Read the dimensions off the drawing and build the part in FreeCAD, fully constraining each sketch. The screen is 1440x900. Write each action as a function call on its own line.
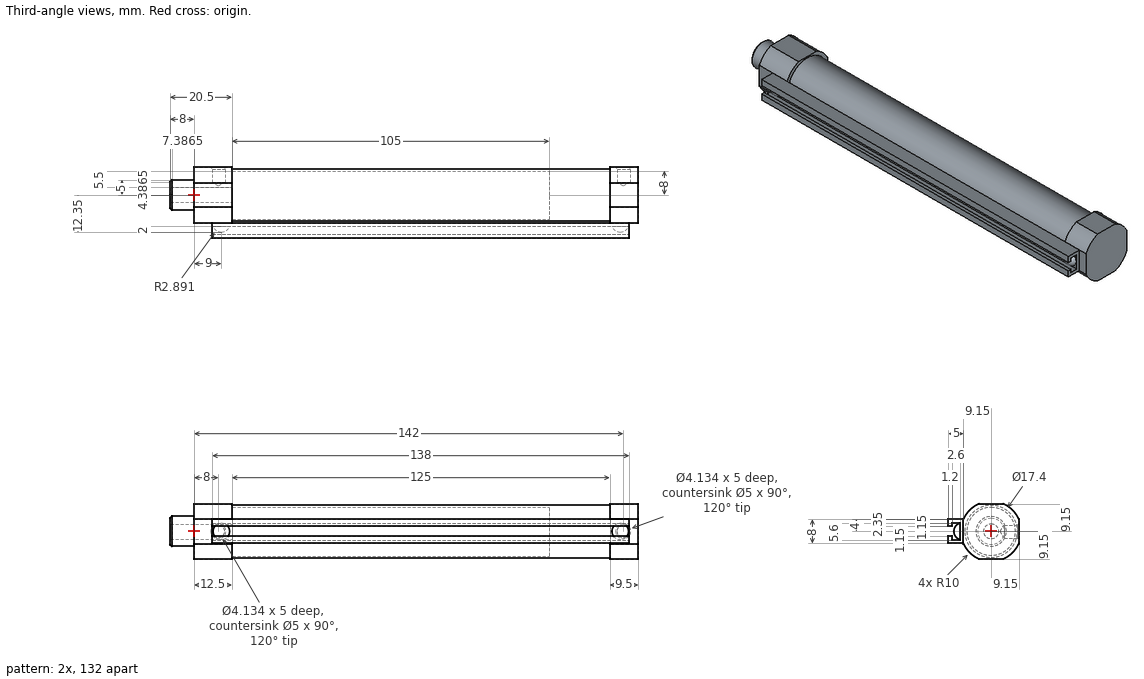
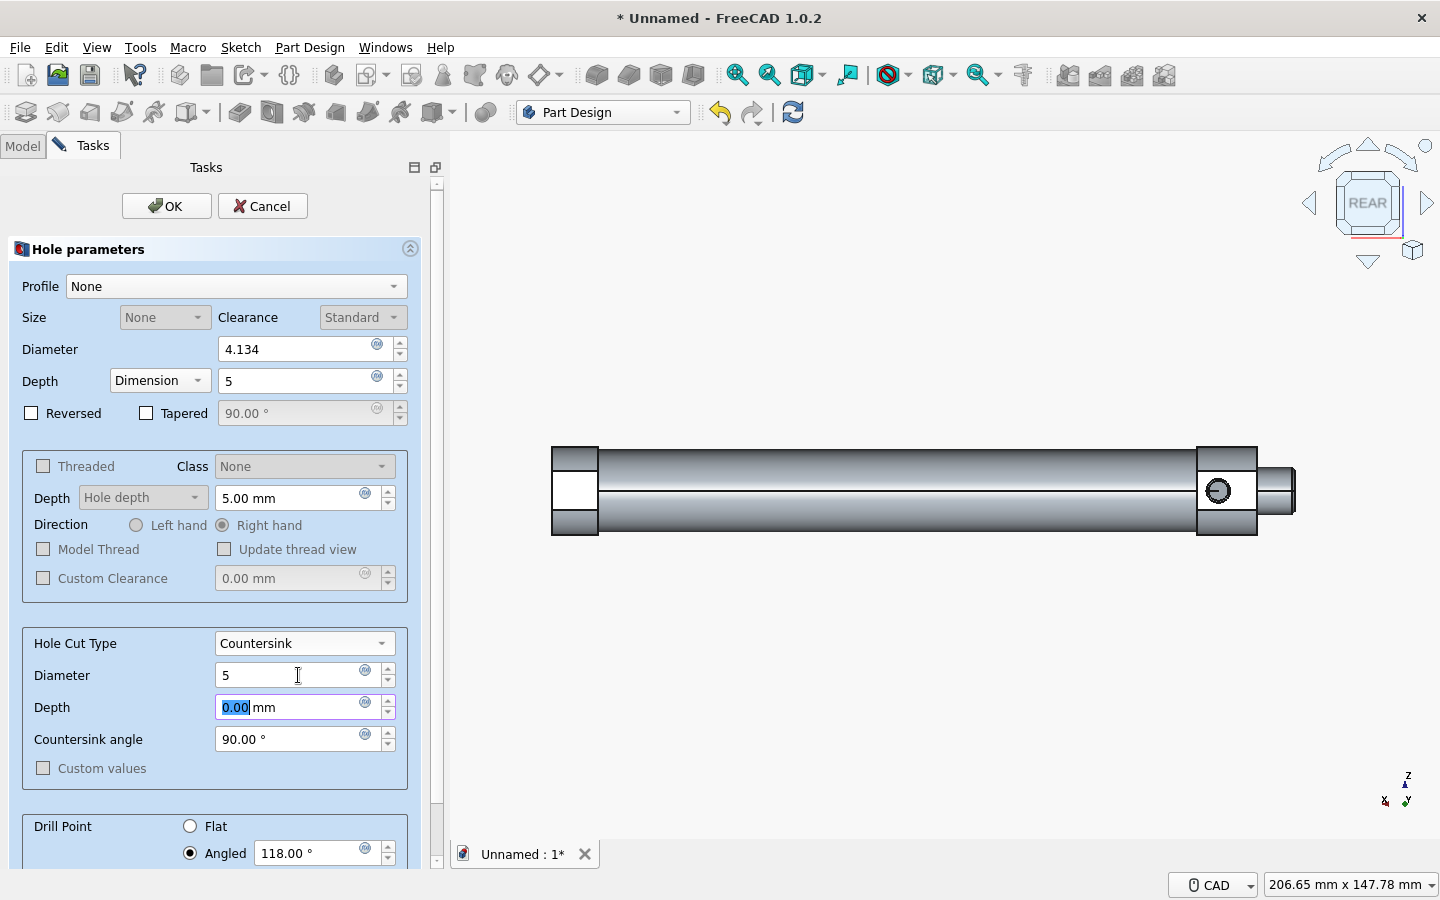
triple_click(317, 853)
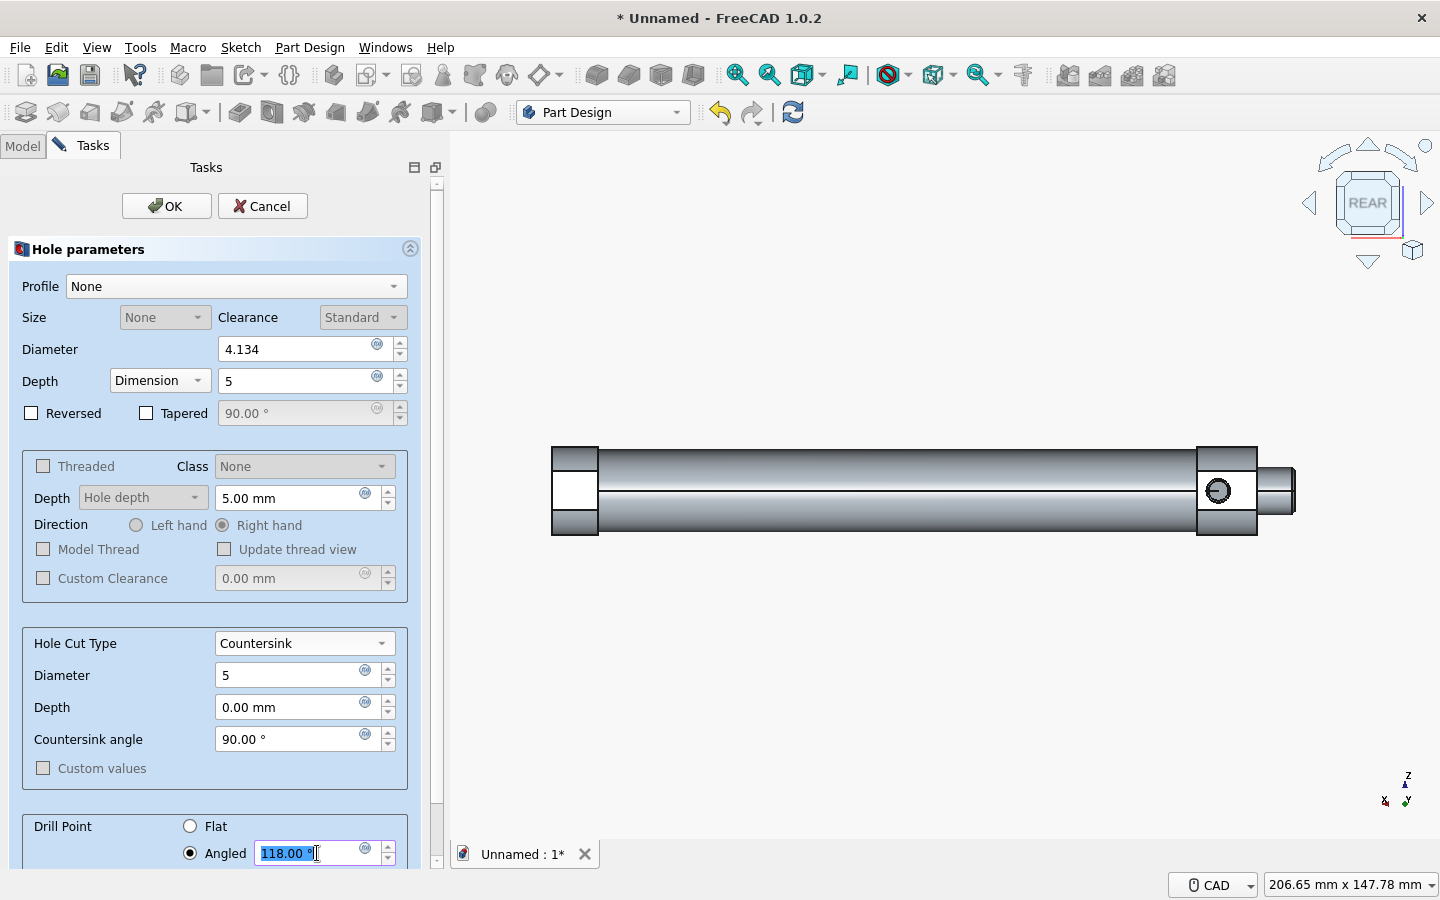
text(120)
key(Tab)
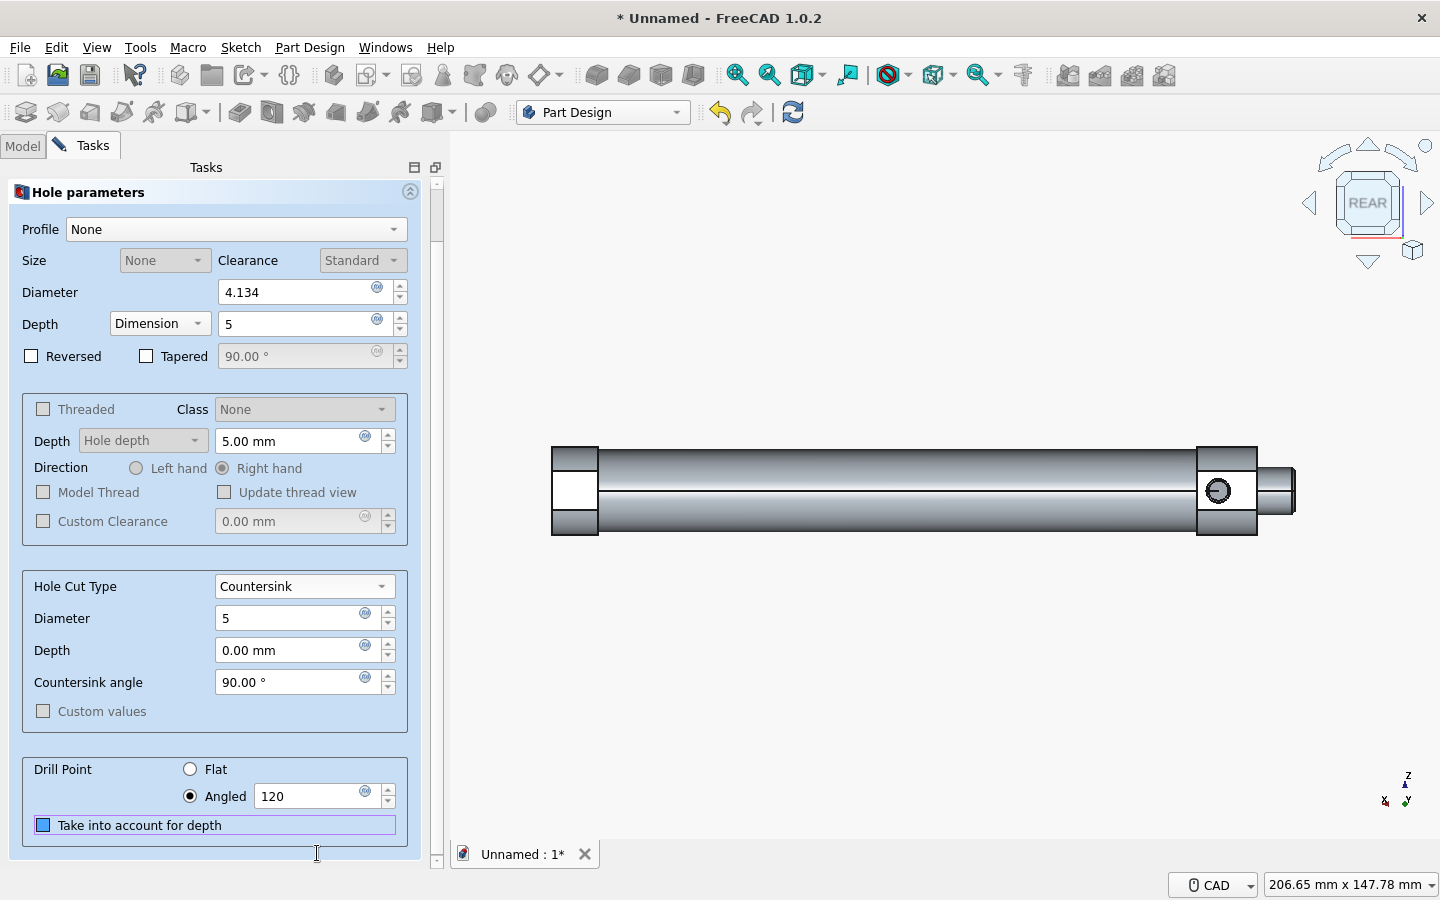
scroll(437, 522, up, 2)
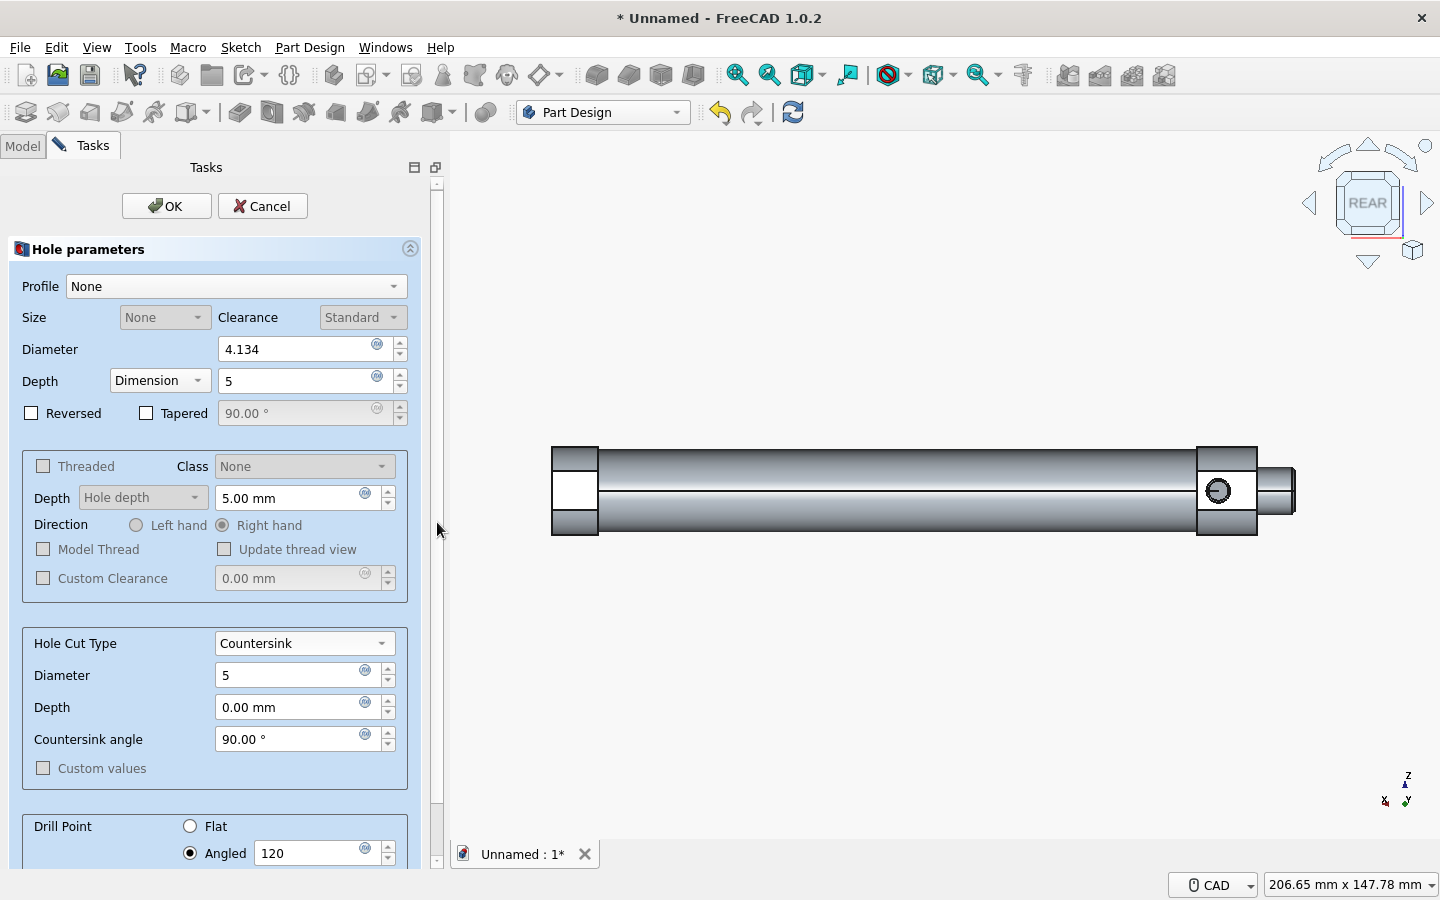
click(167, 206)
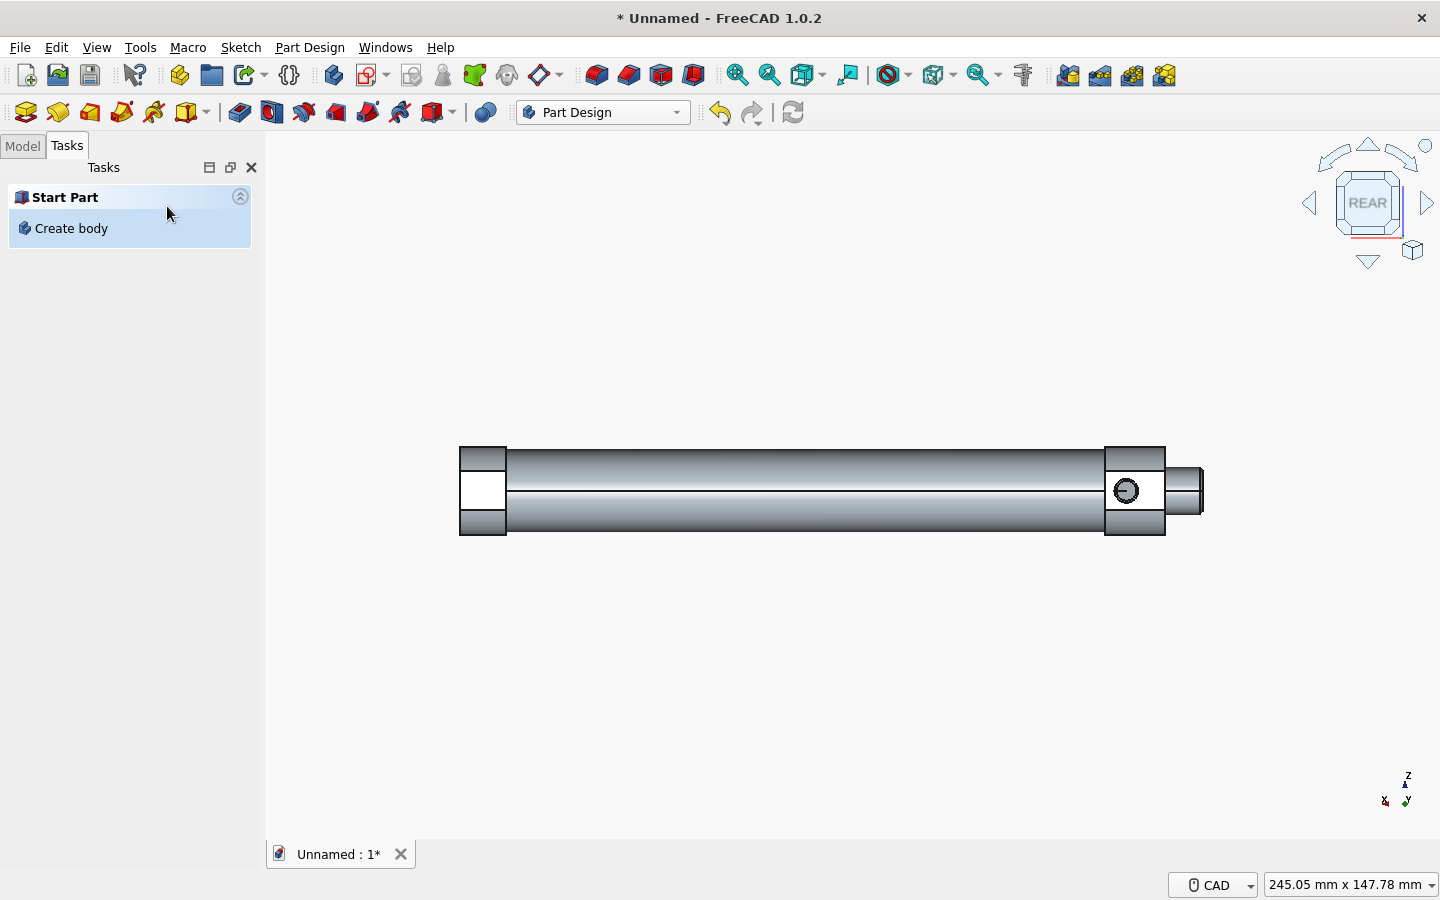
click(1152, 484)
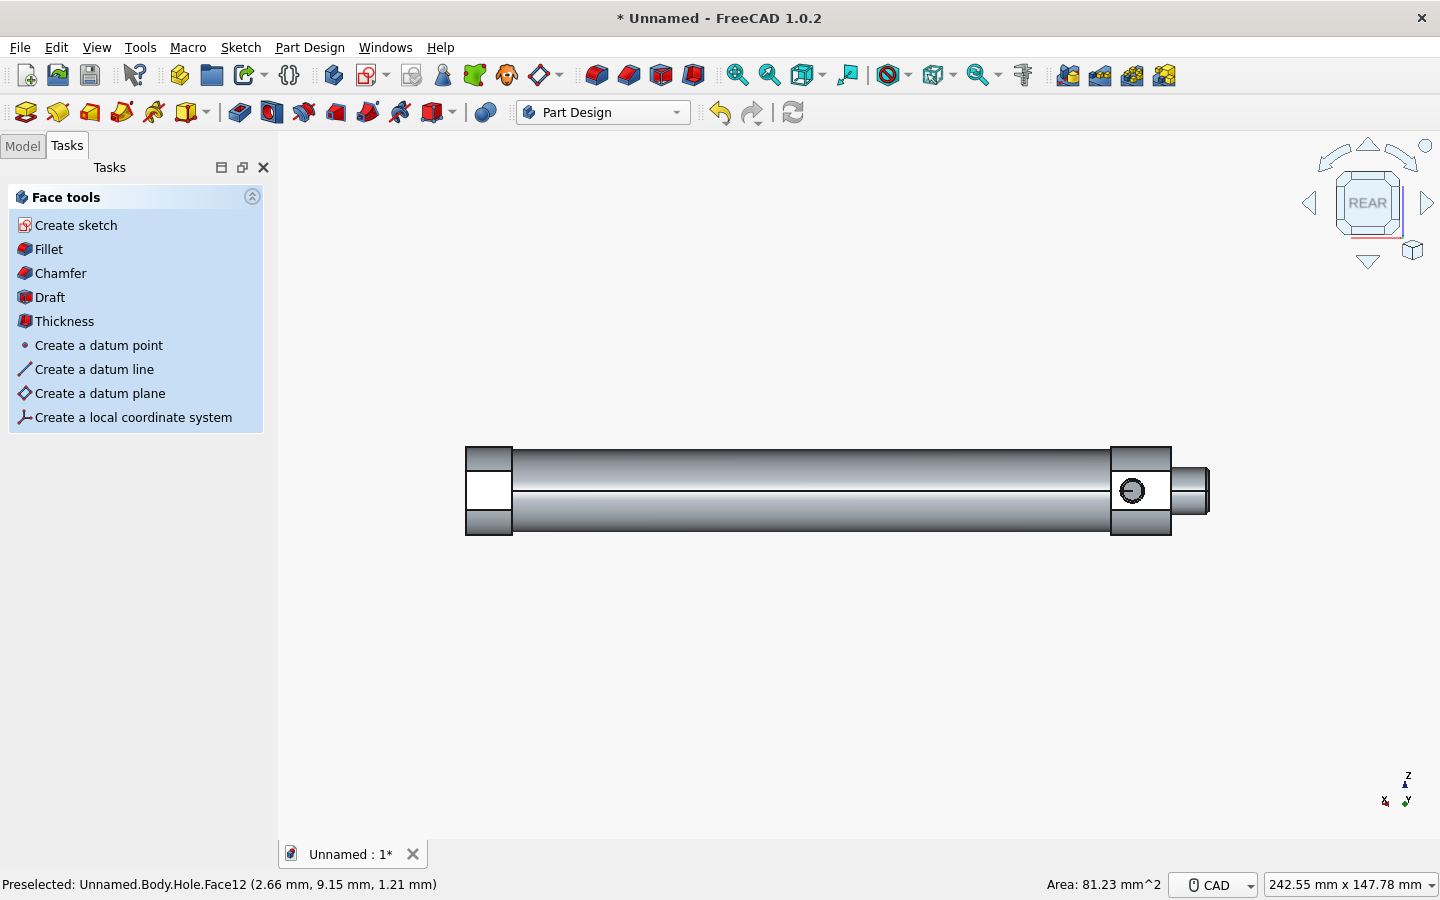
click(366, 76)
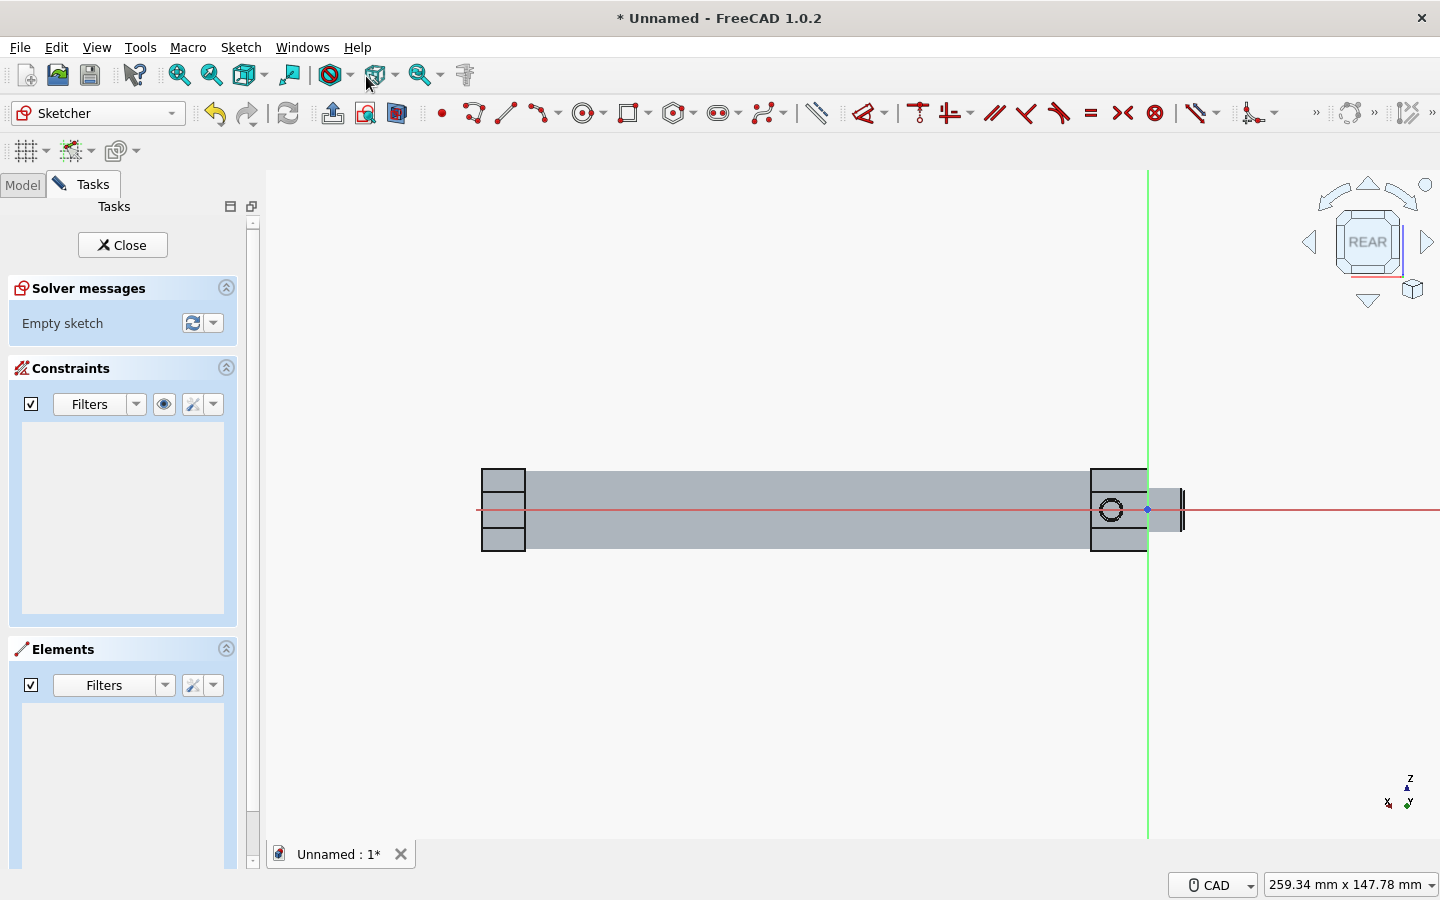
scroll(490, 510, up, 15)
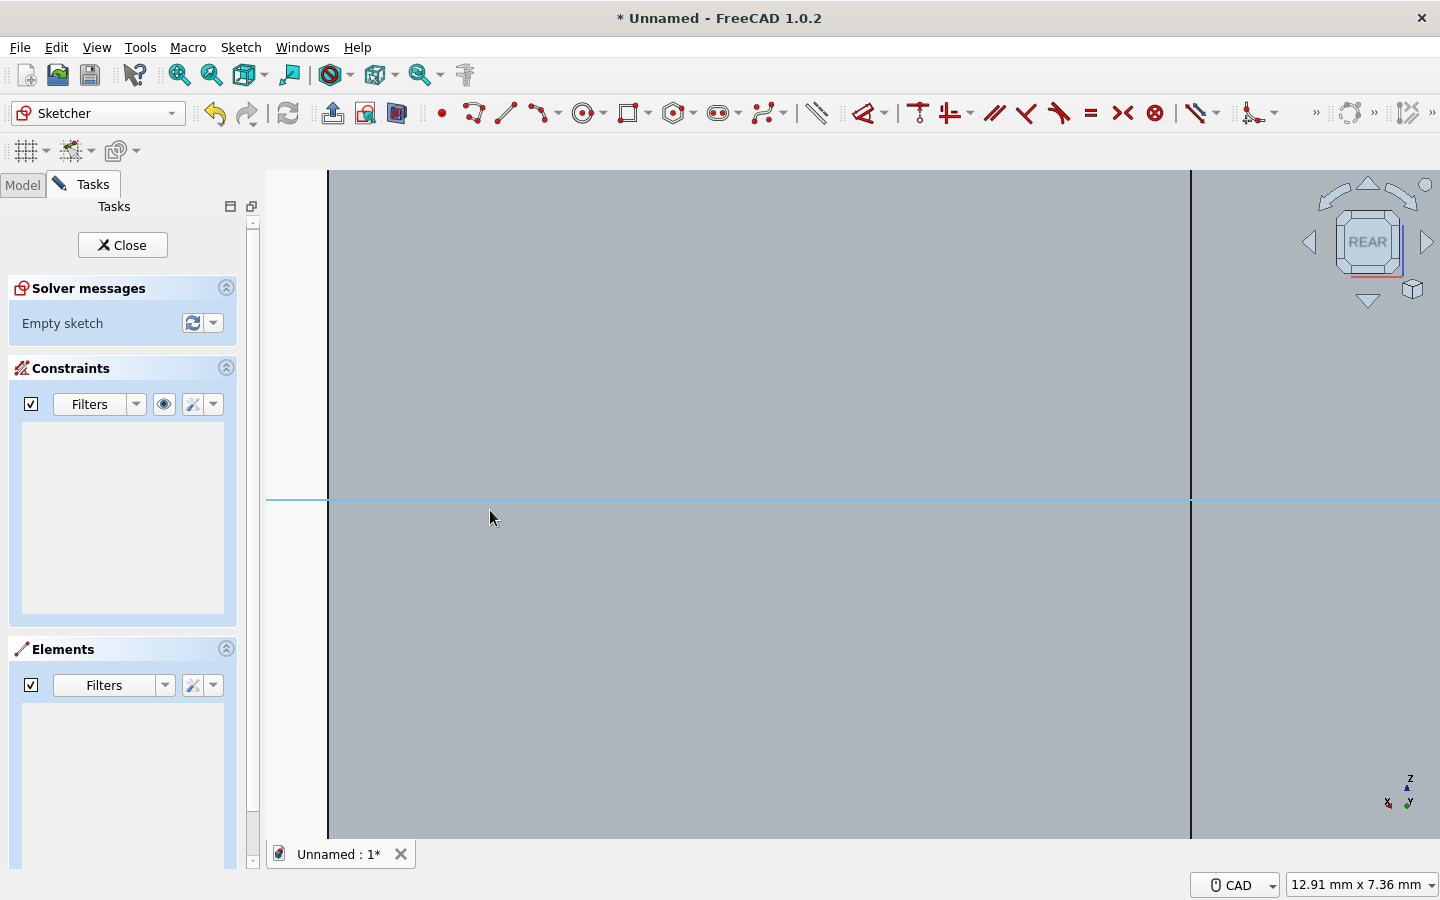
click(584, 114)